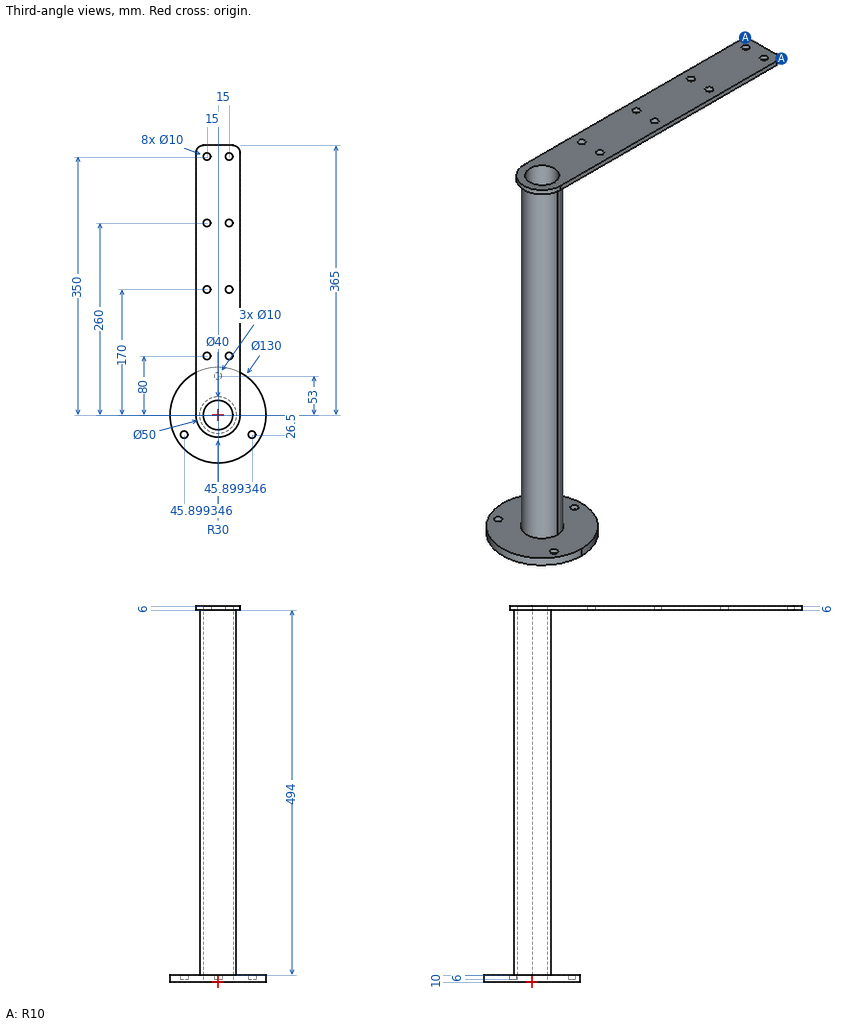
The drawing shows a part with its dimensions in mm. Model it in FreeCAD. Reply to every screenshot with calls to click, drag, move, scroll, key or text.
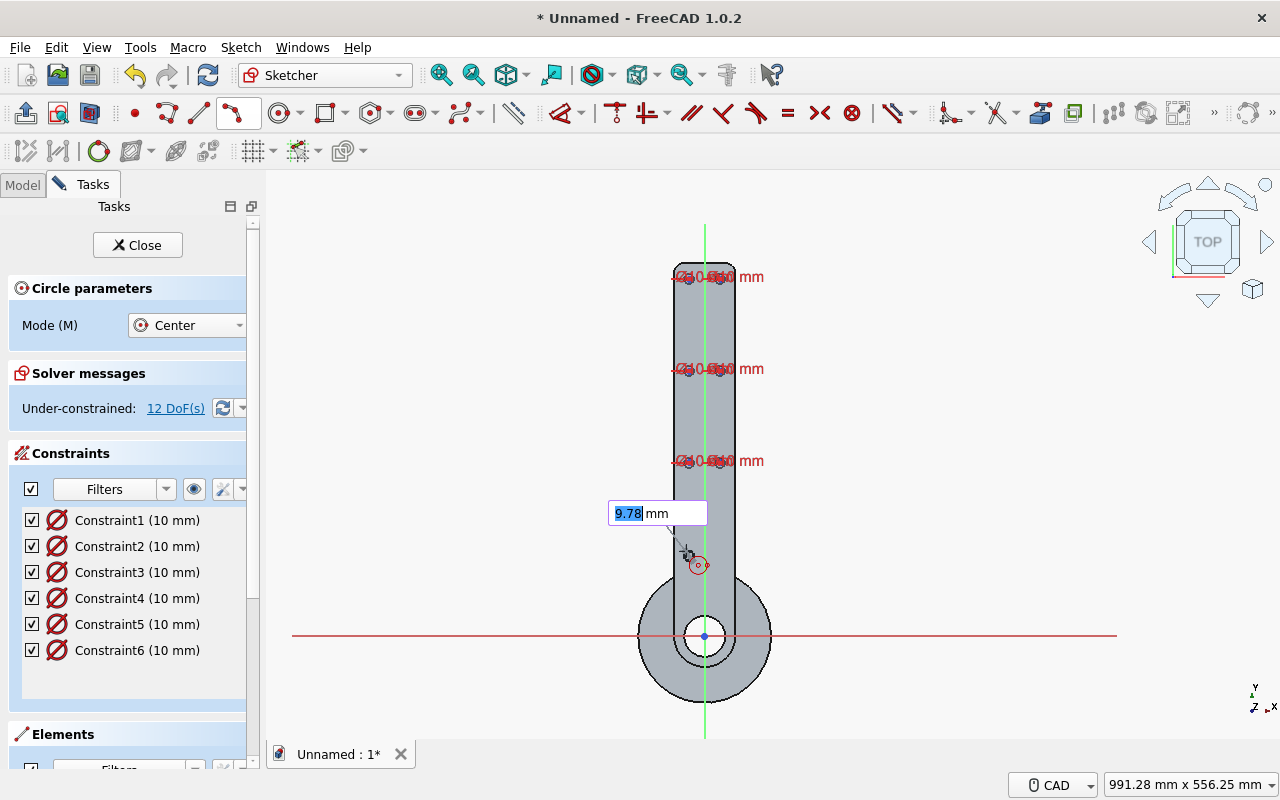
text(10)
key(Return)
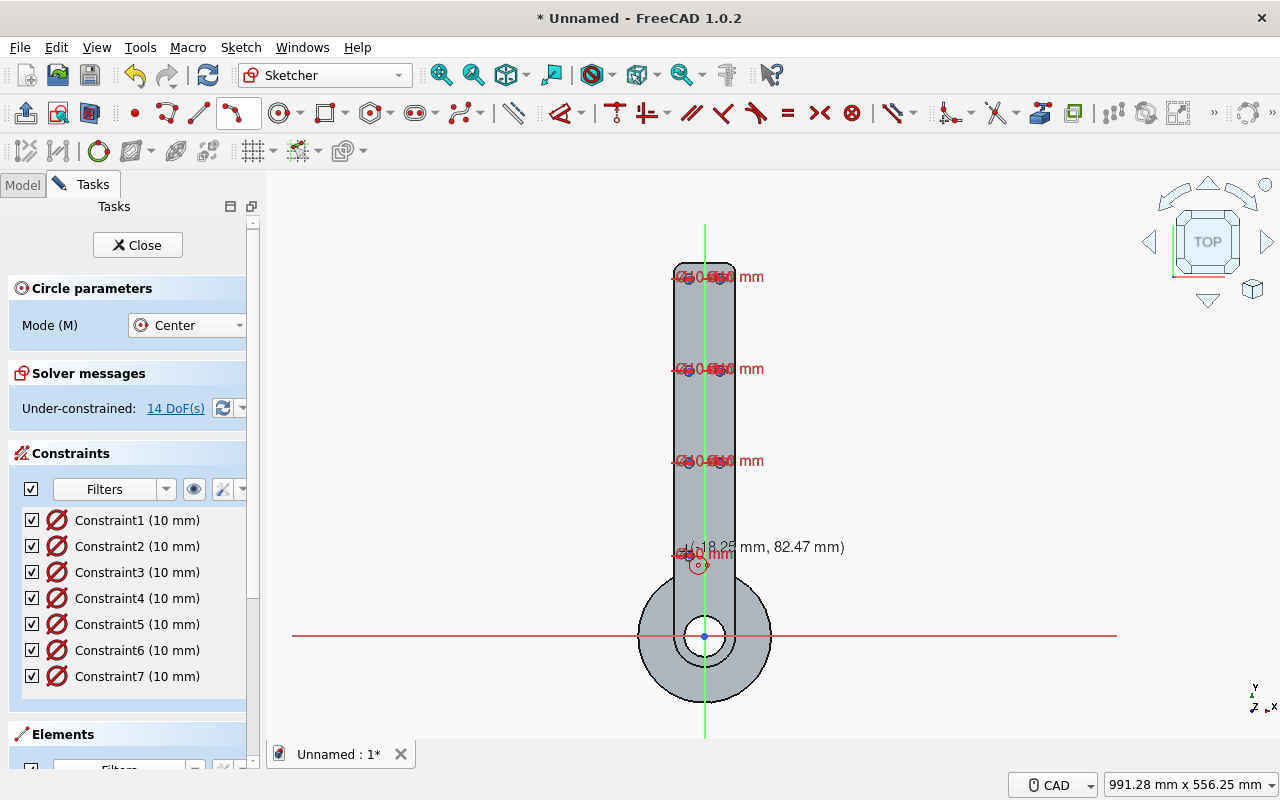
scroll(720, 555, up, 8)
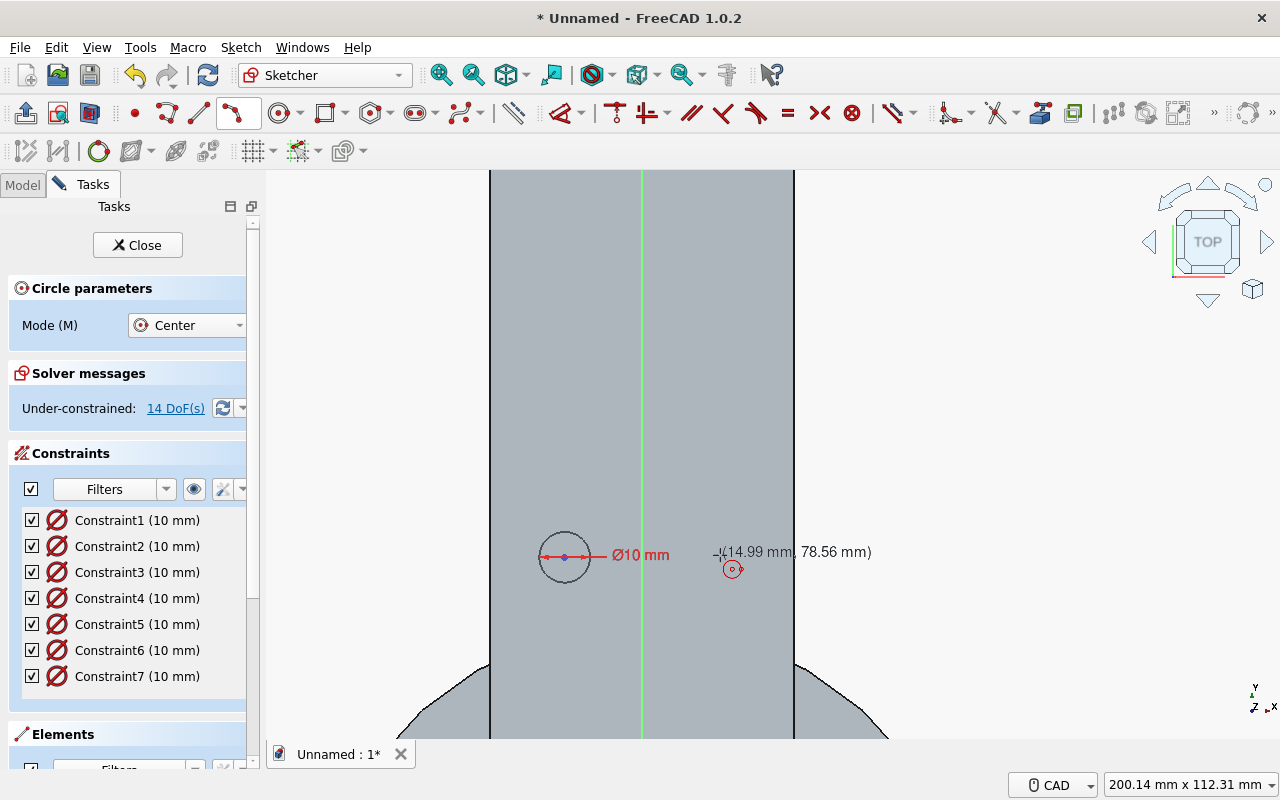
scroll(720, 555, down, 8)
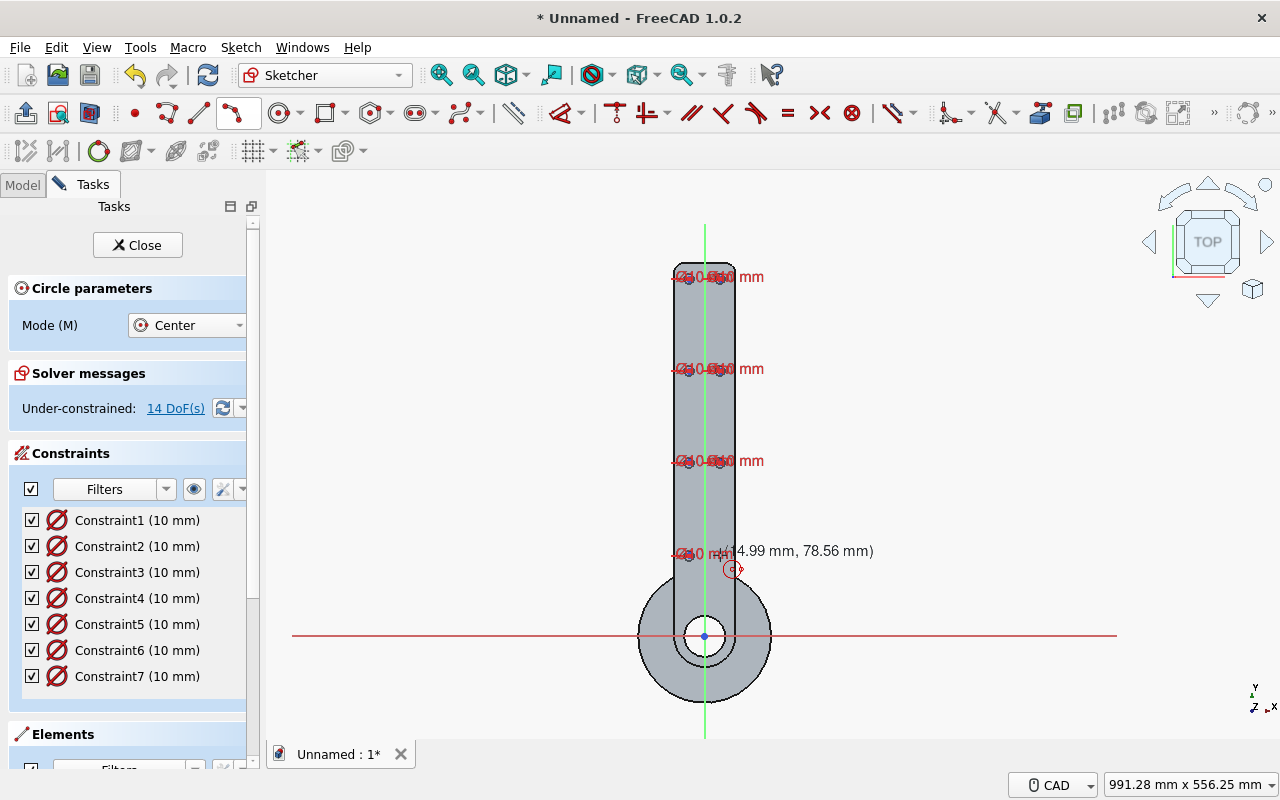
click(720, 555)
move(724, 551)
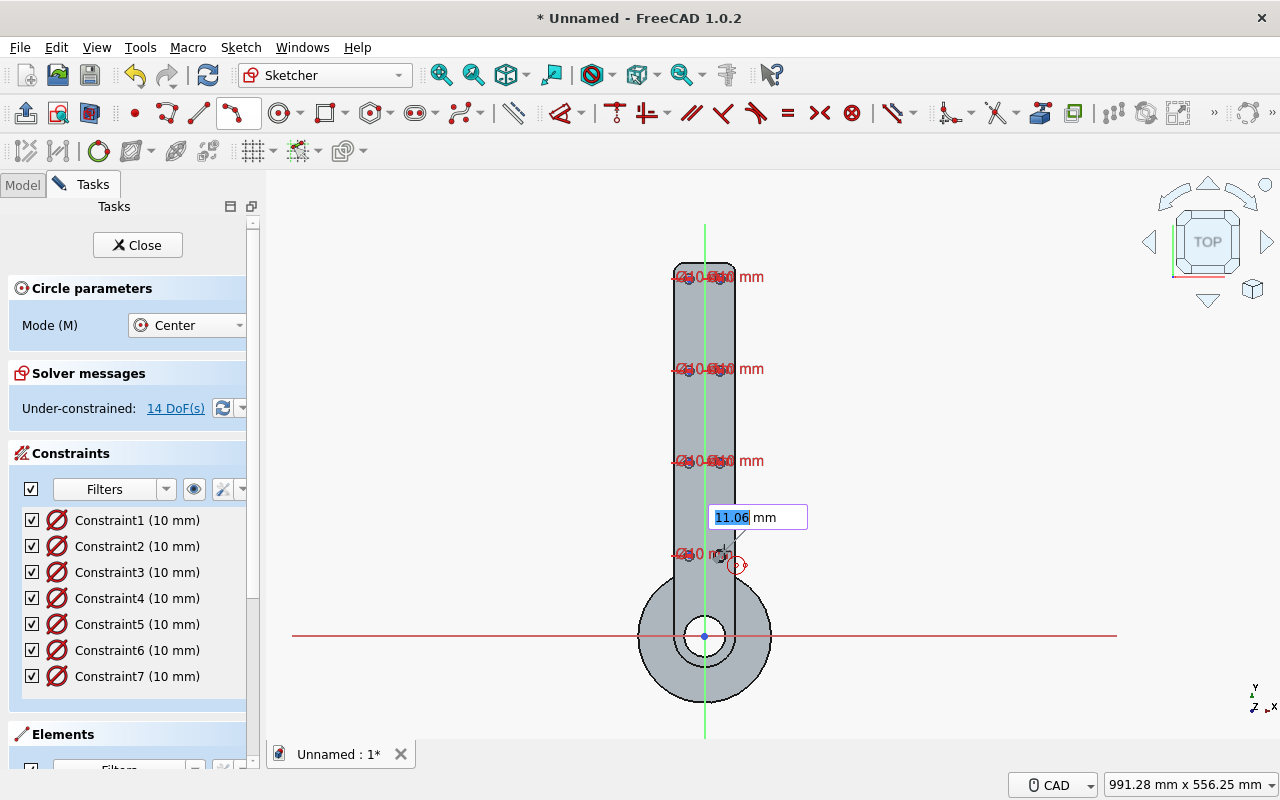
text(10)
key(Return)
key(Escape)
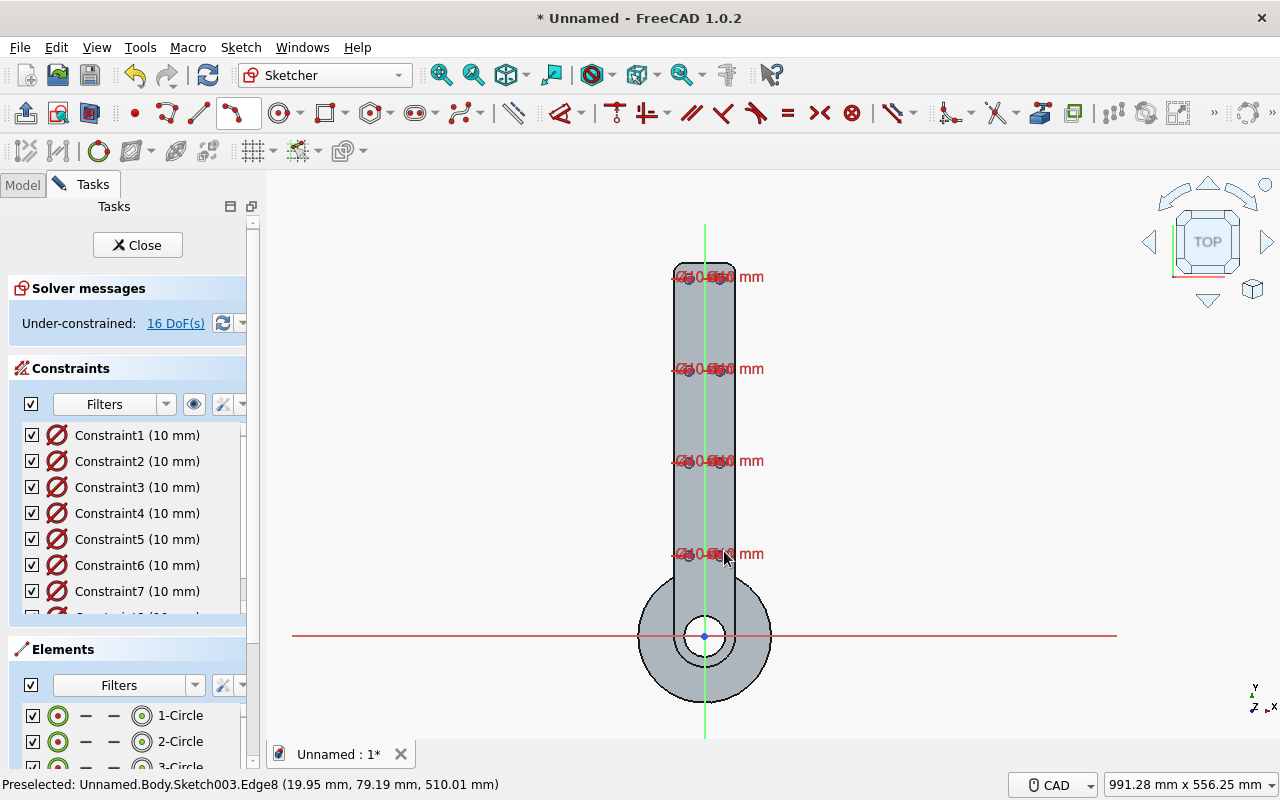
click(689, 279)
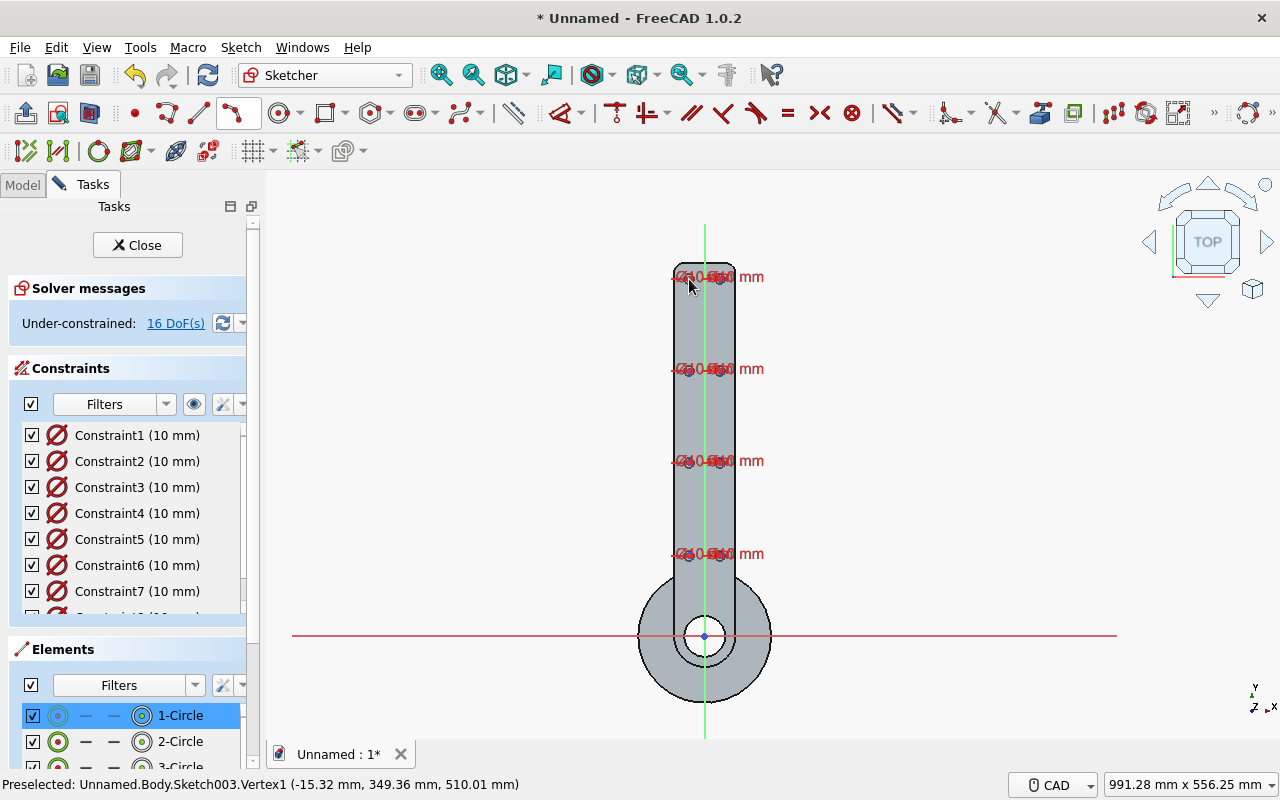
click(720, 279)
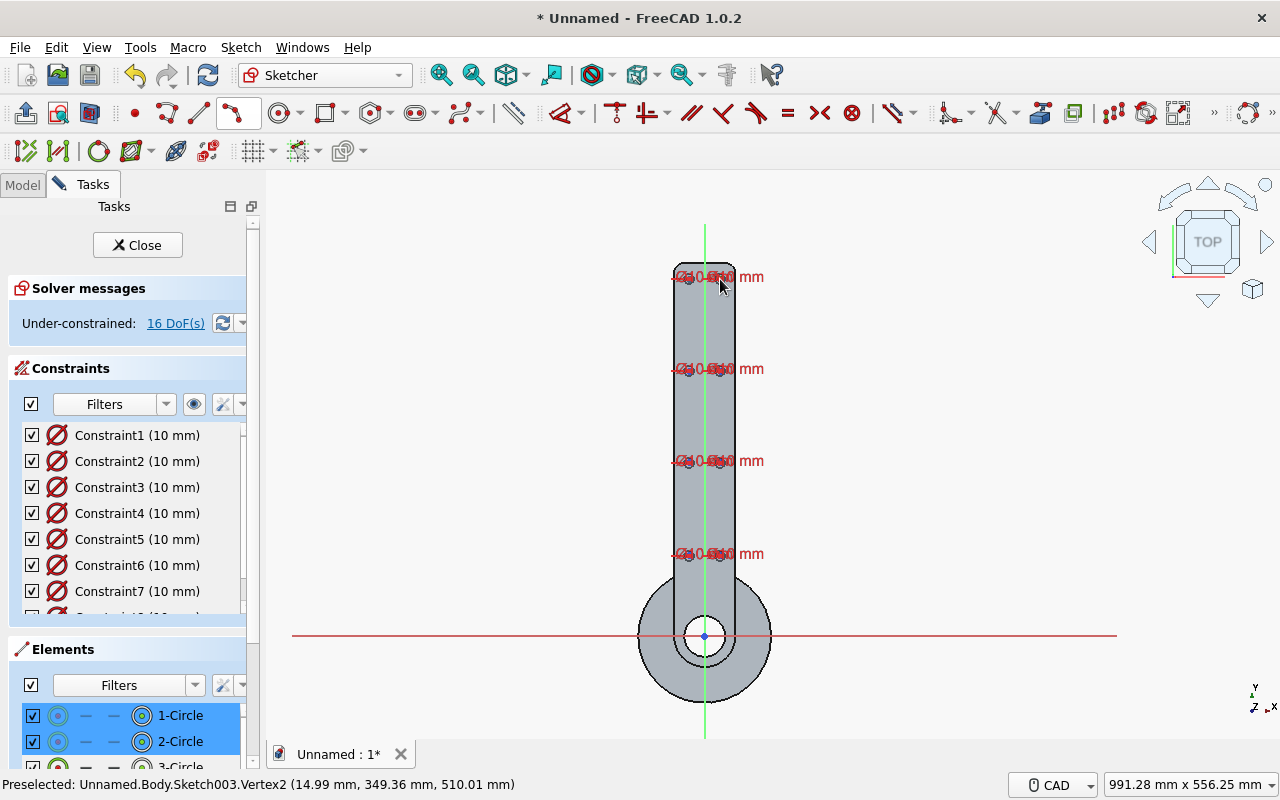
click(670, 114)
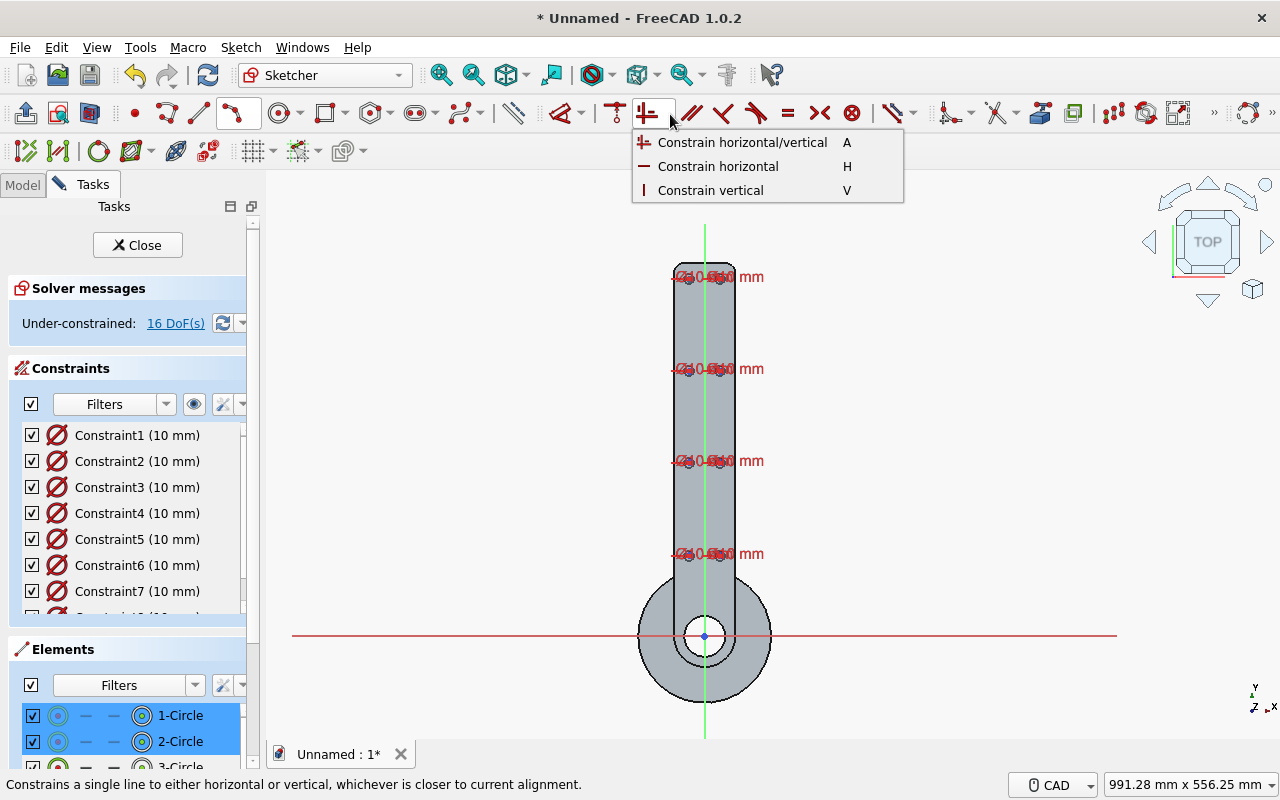
click(768, 166)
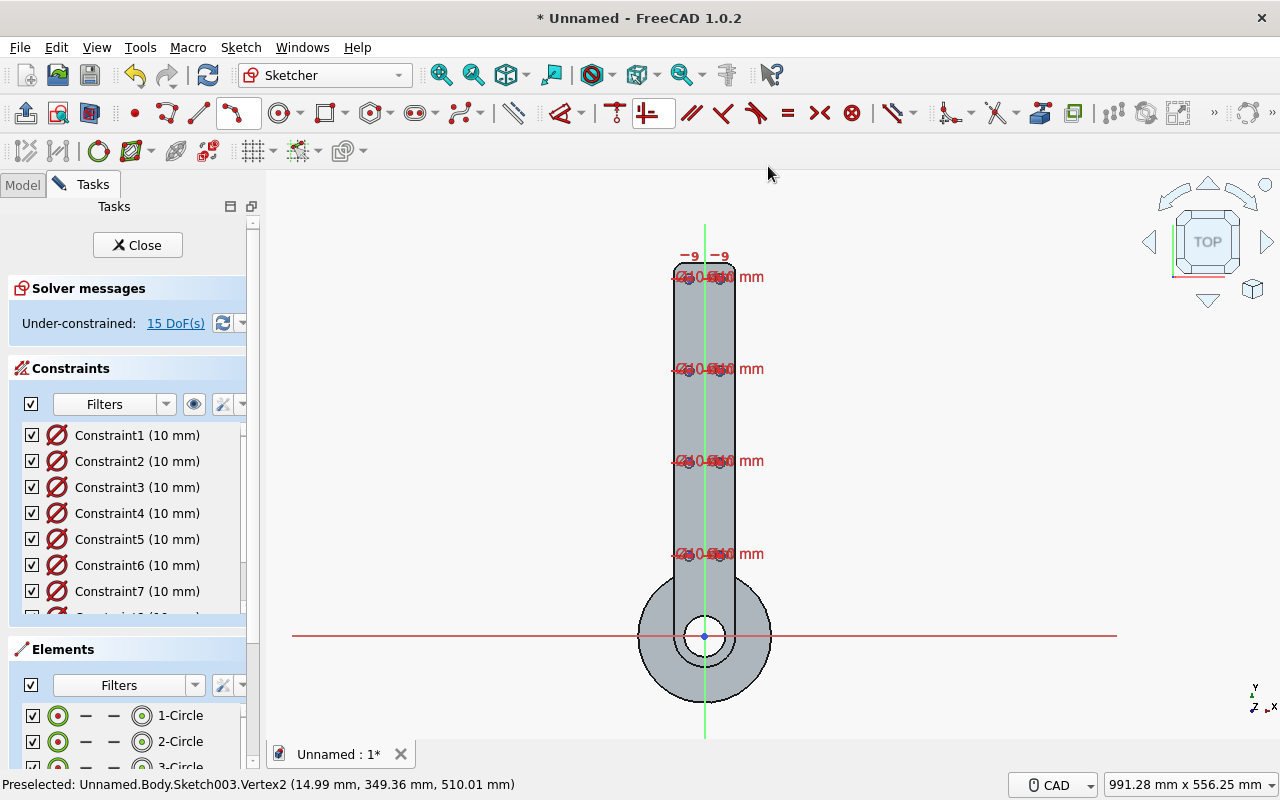
click(689, 279)